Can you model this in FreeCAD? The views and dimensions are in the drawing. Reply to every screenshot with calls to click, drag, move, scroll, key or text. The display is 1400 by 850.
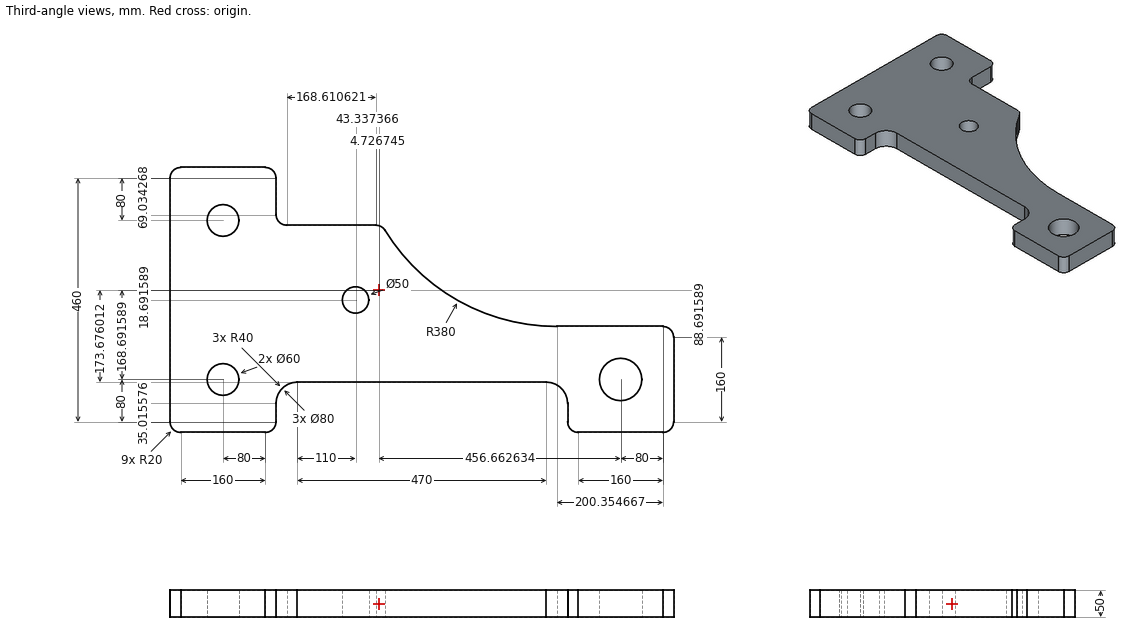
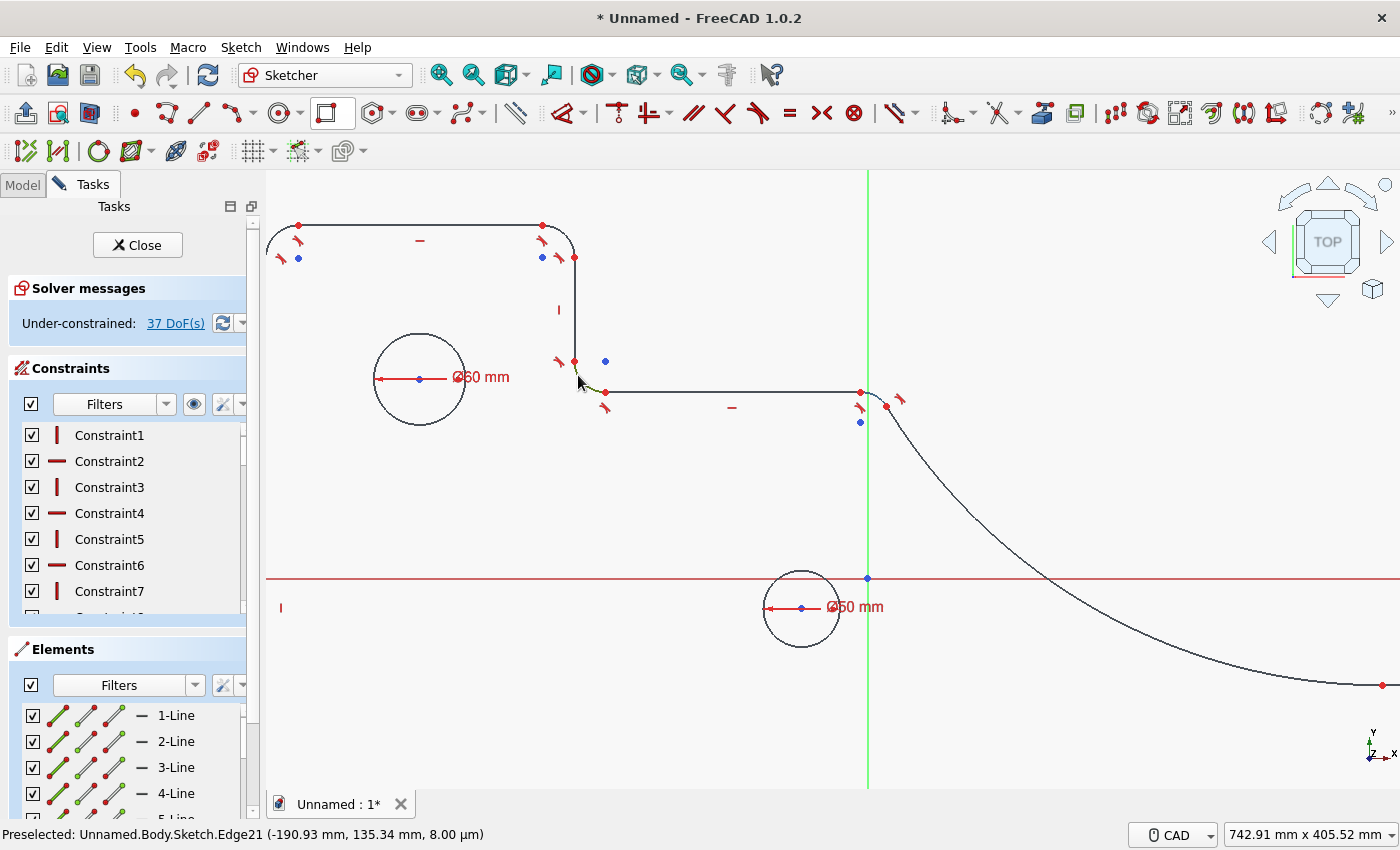
click(571, 243)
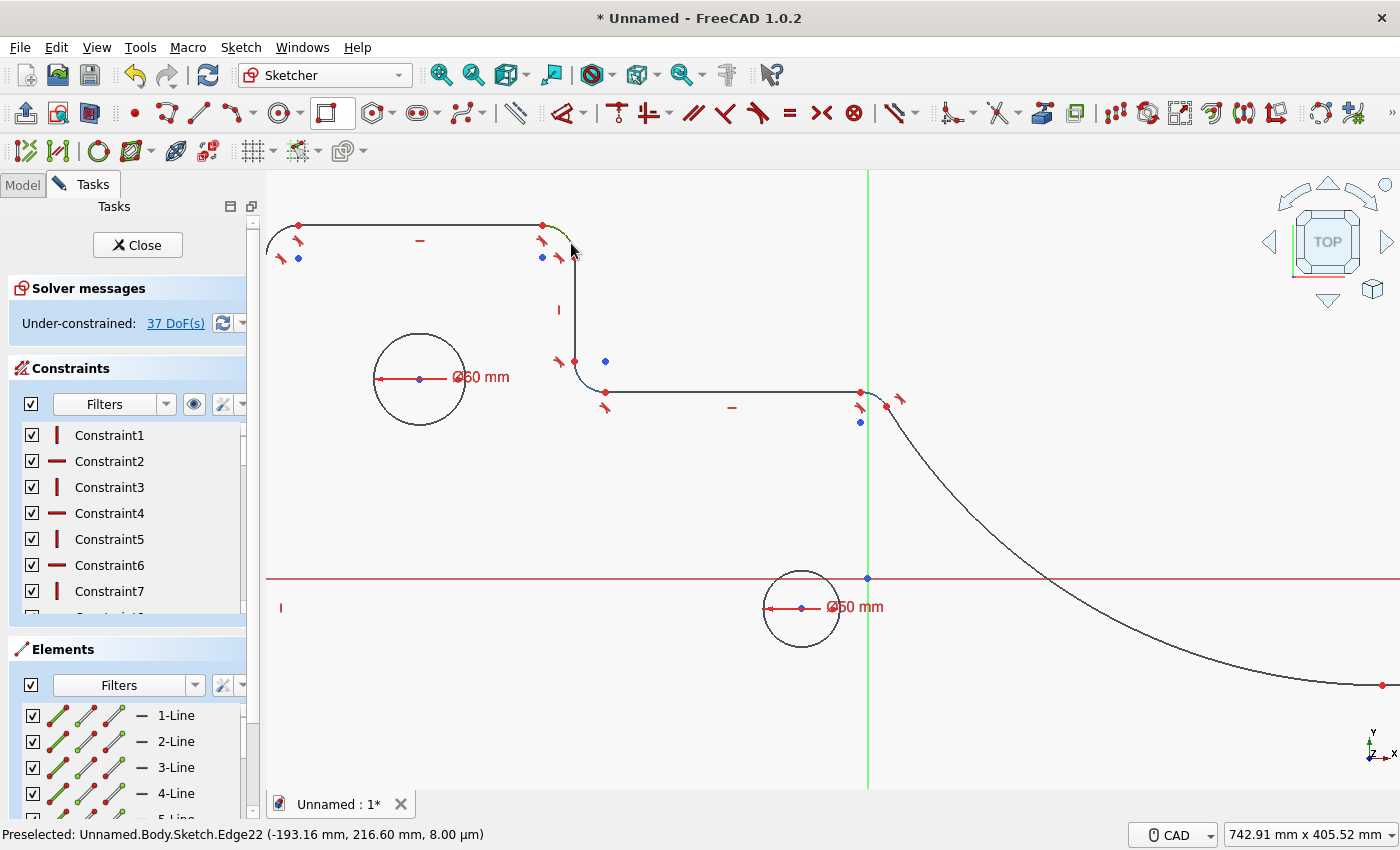
scroll(578, 375, down, 4)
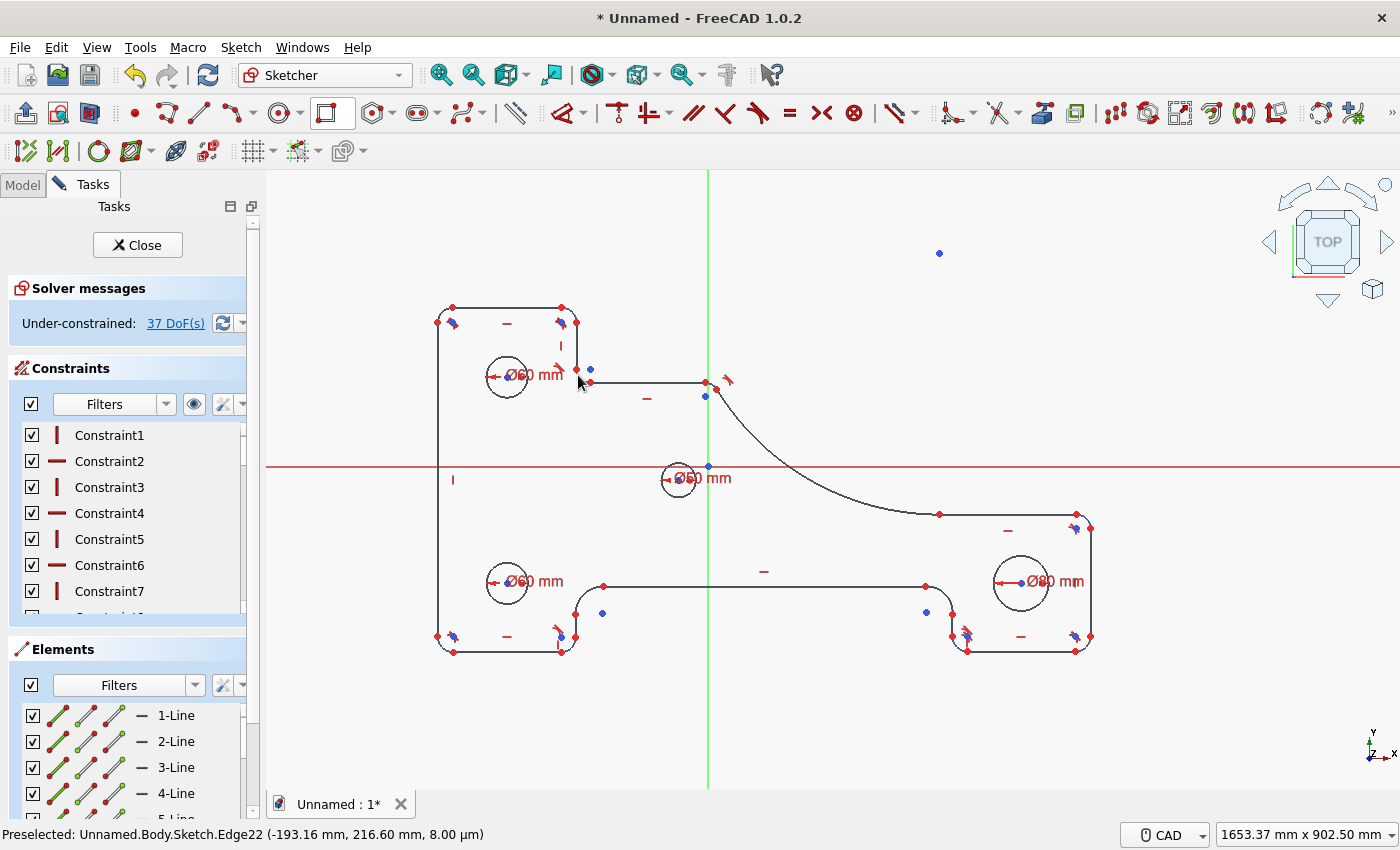
scroll(446, 310, up, 4)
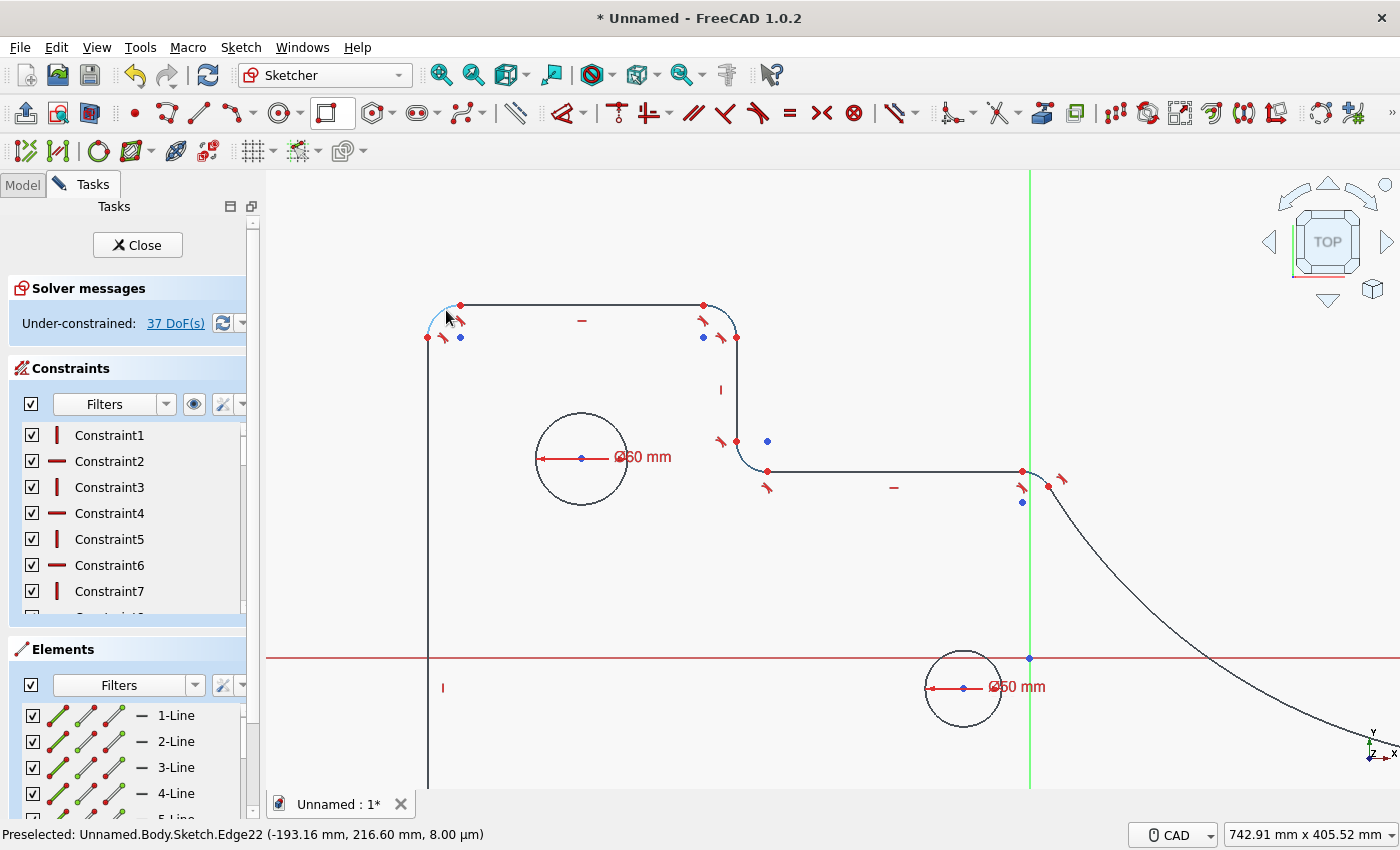
click(446, 309)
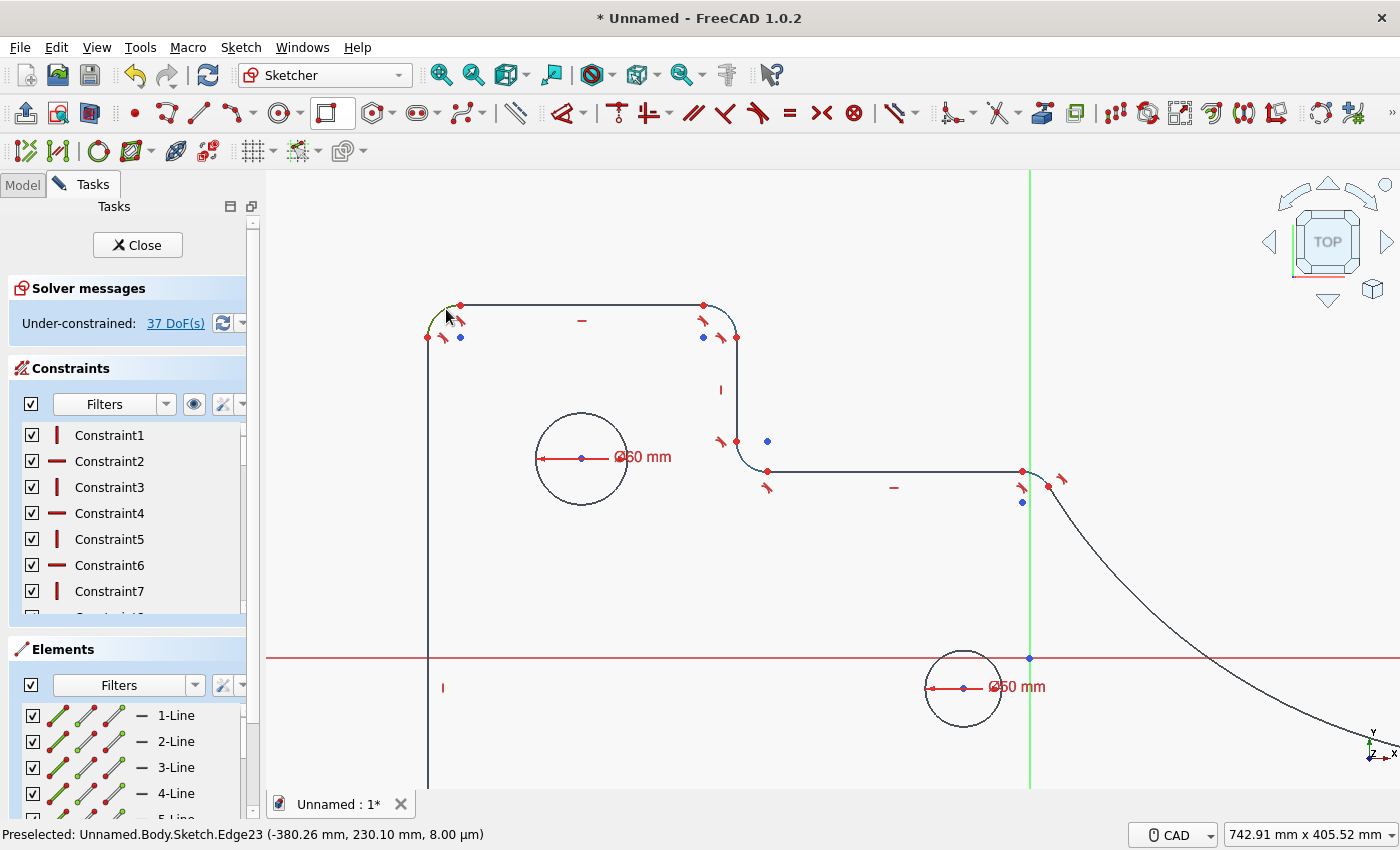
click(790, 114)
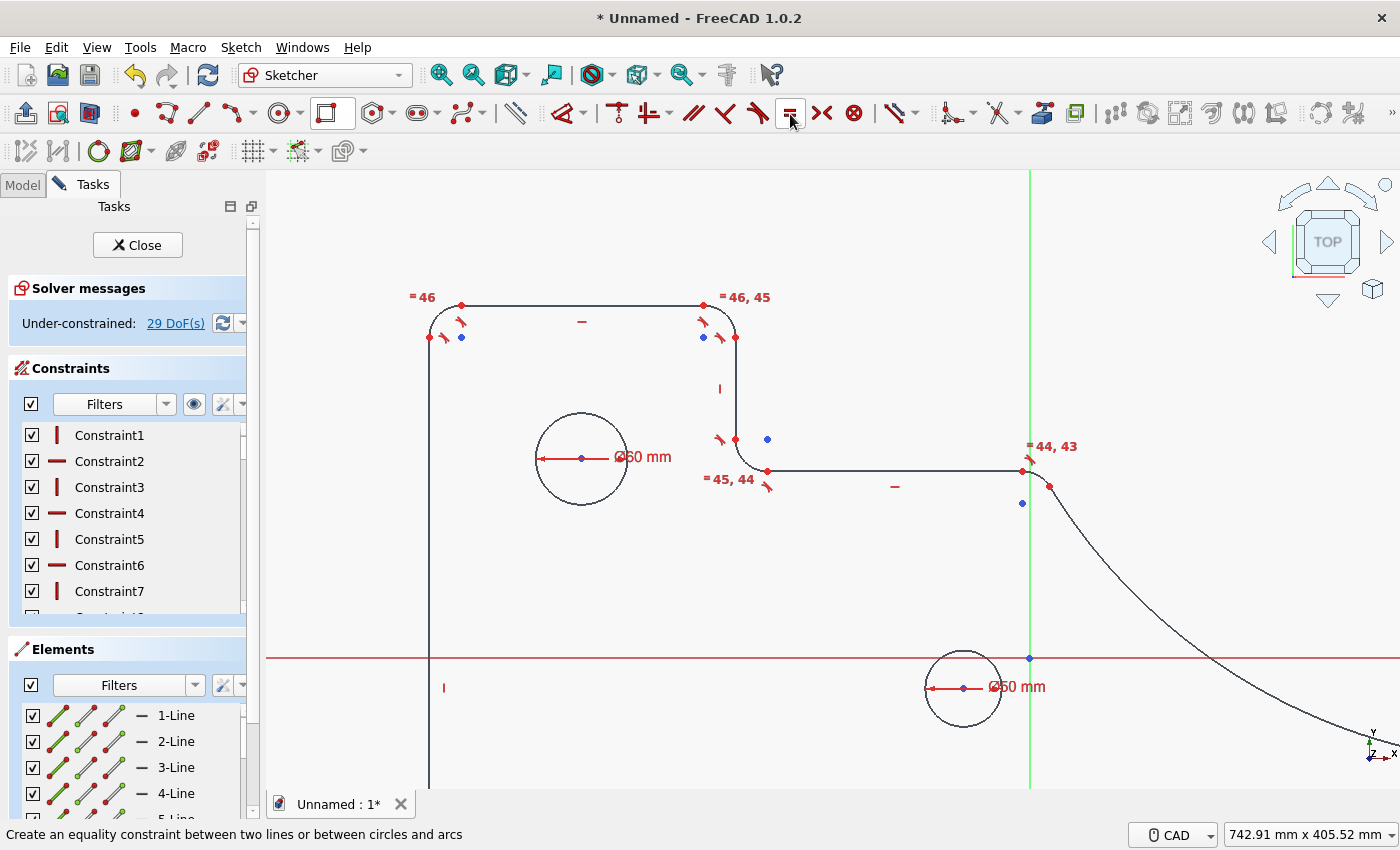
scroll(446, 310, down, 4)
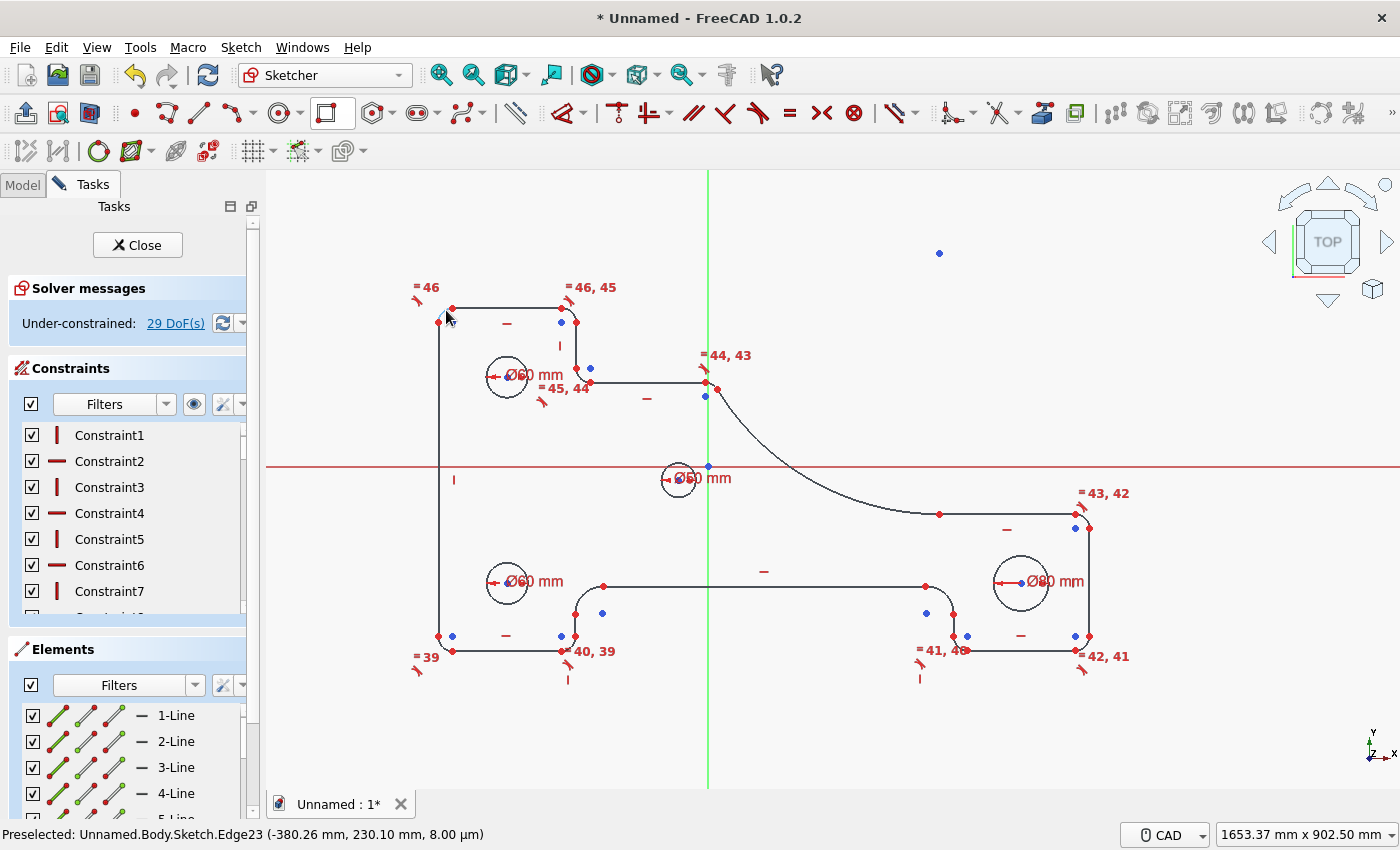
click(591, 589)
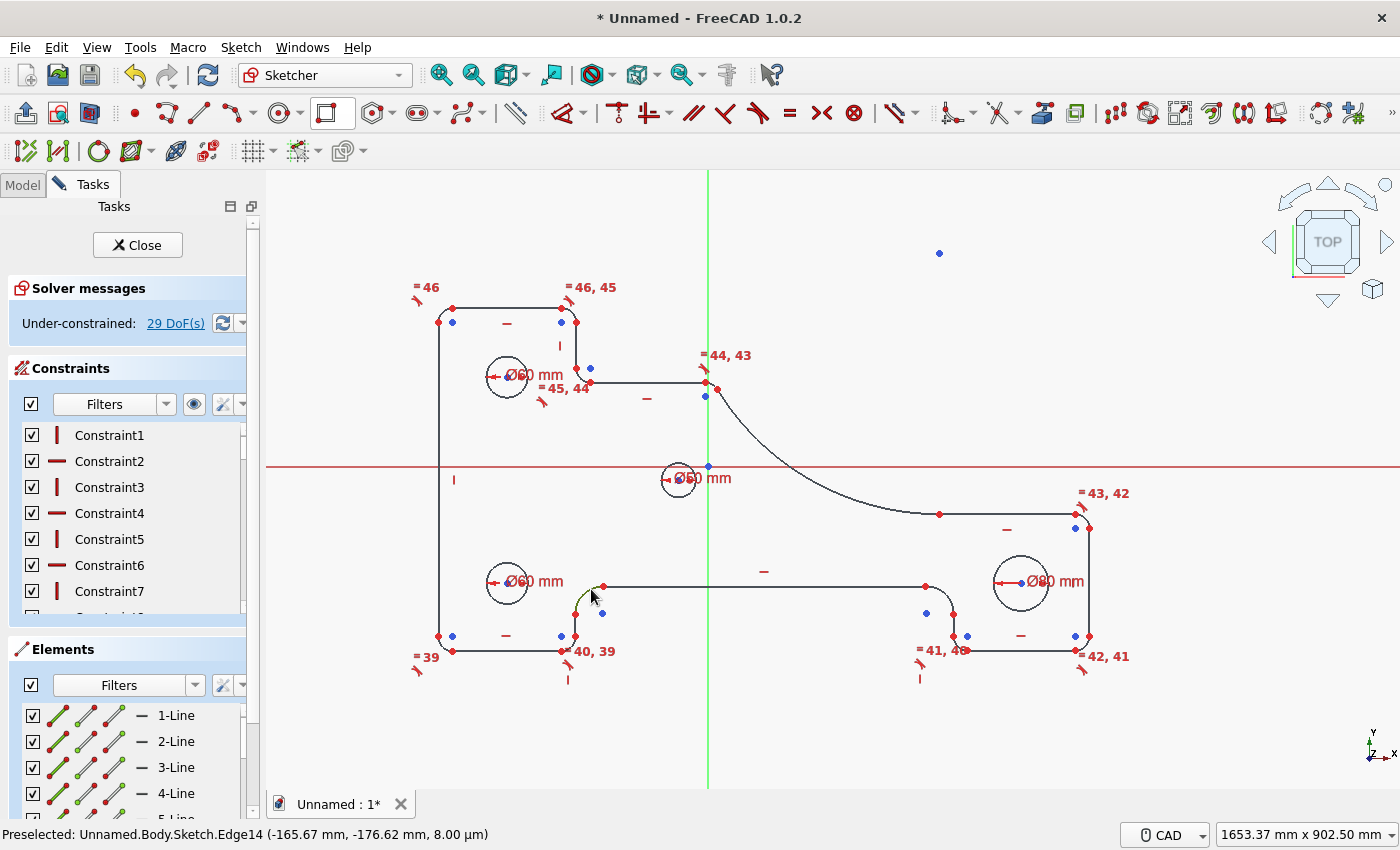
click(951, 602)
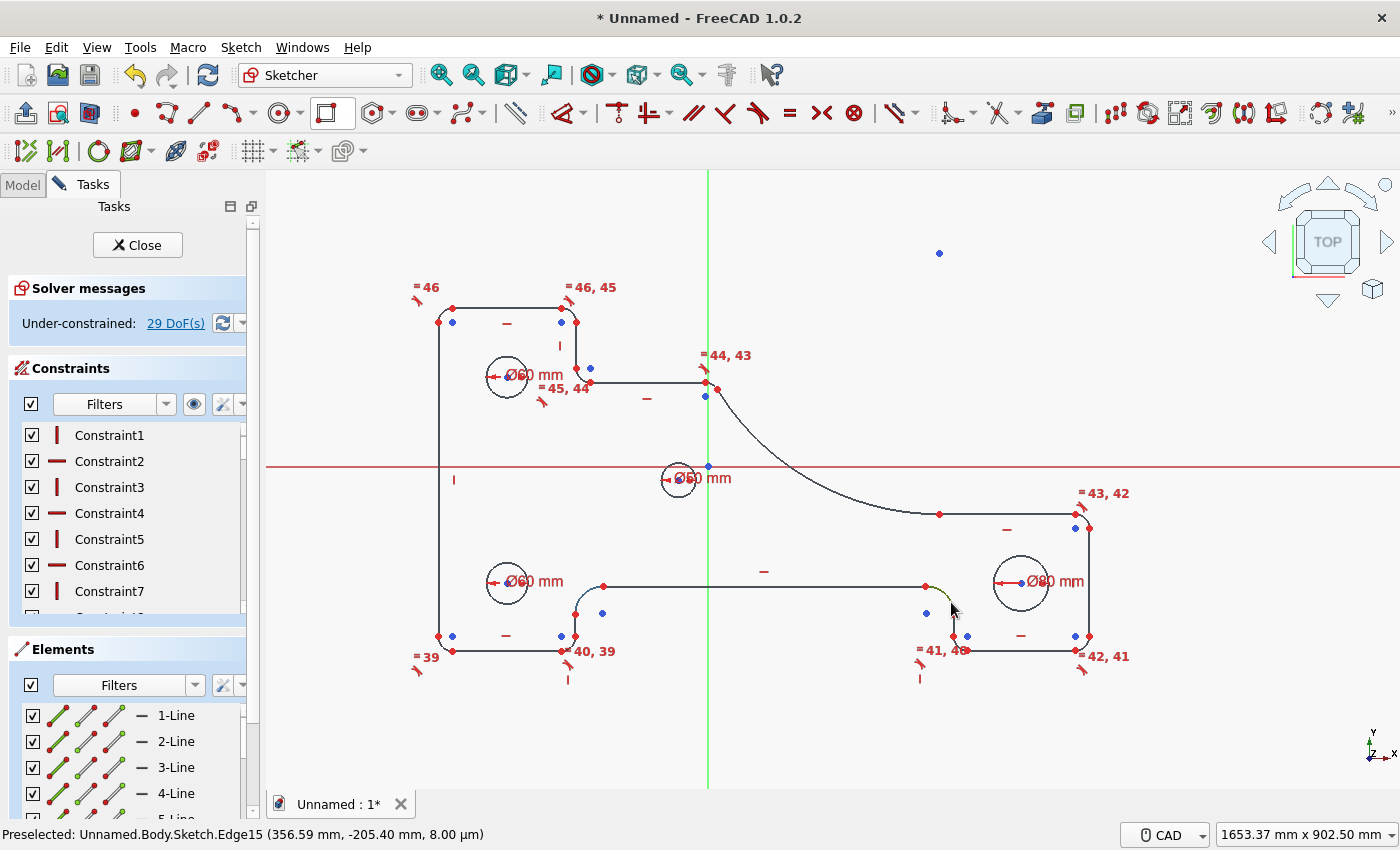
click(790, 114)